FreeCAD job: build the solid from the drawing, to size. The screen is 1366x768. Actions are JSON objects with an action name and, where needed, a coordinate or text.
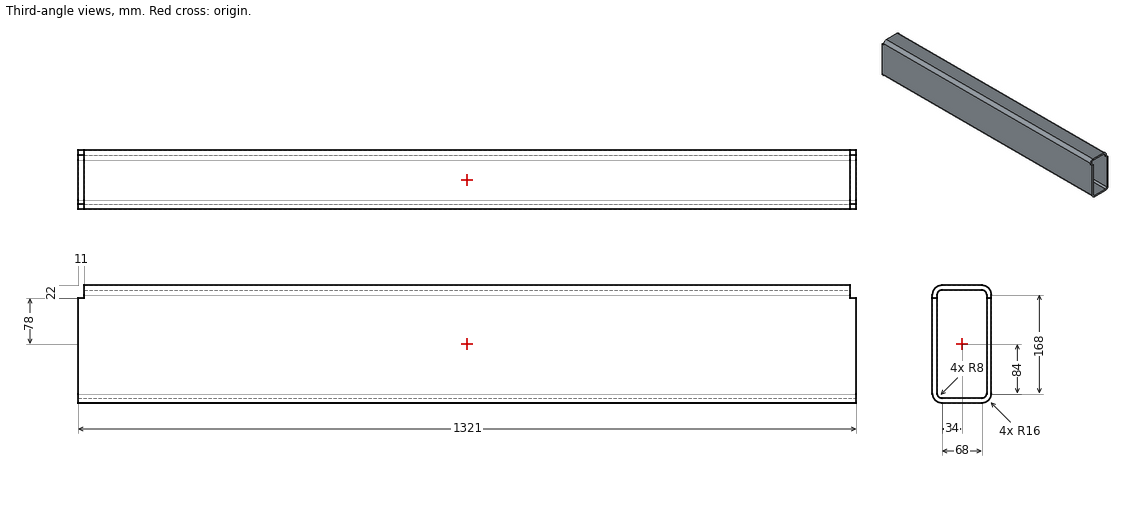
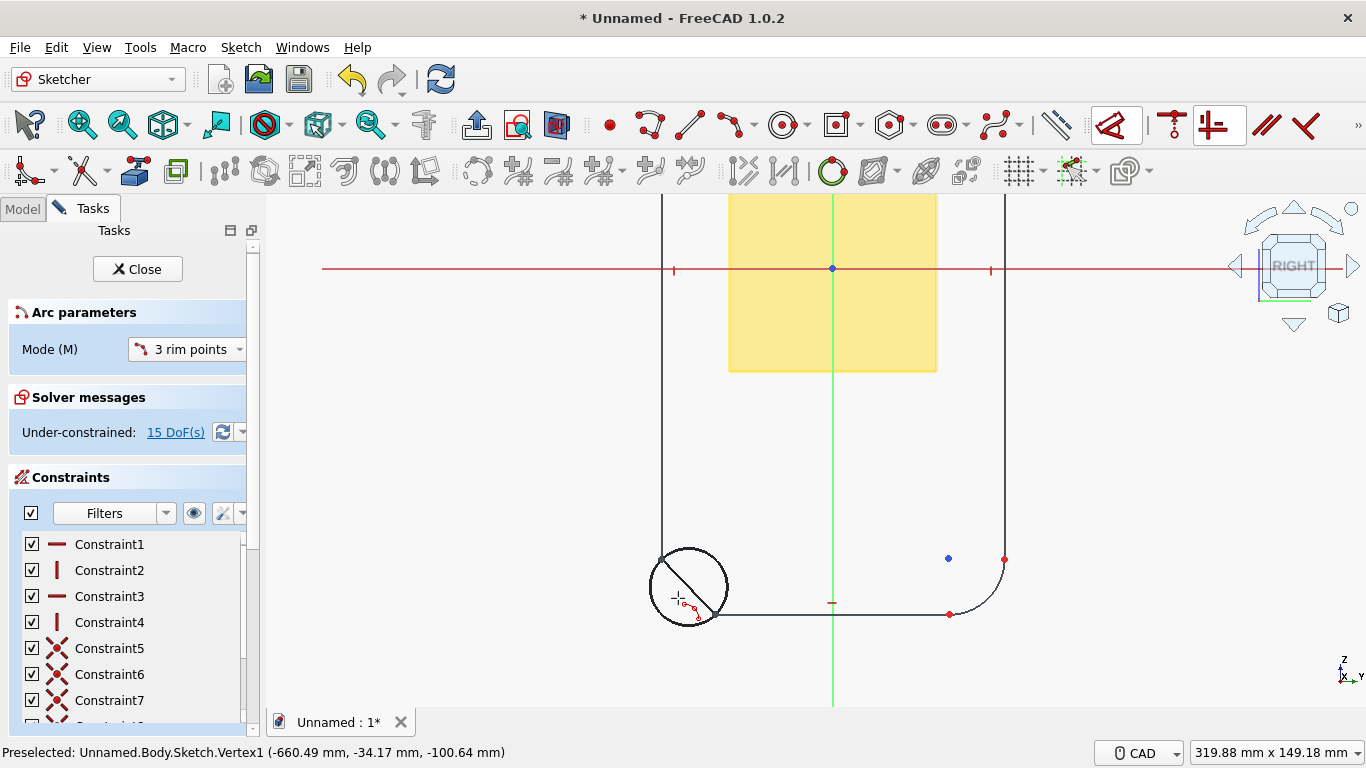
{"action": "left_click", "coordinate": [677, 597]}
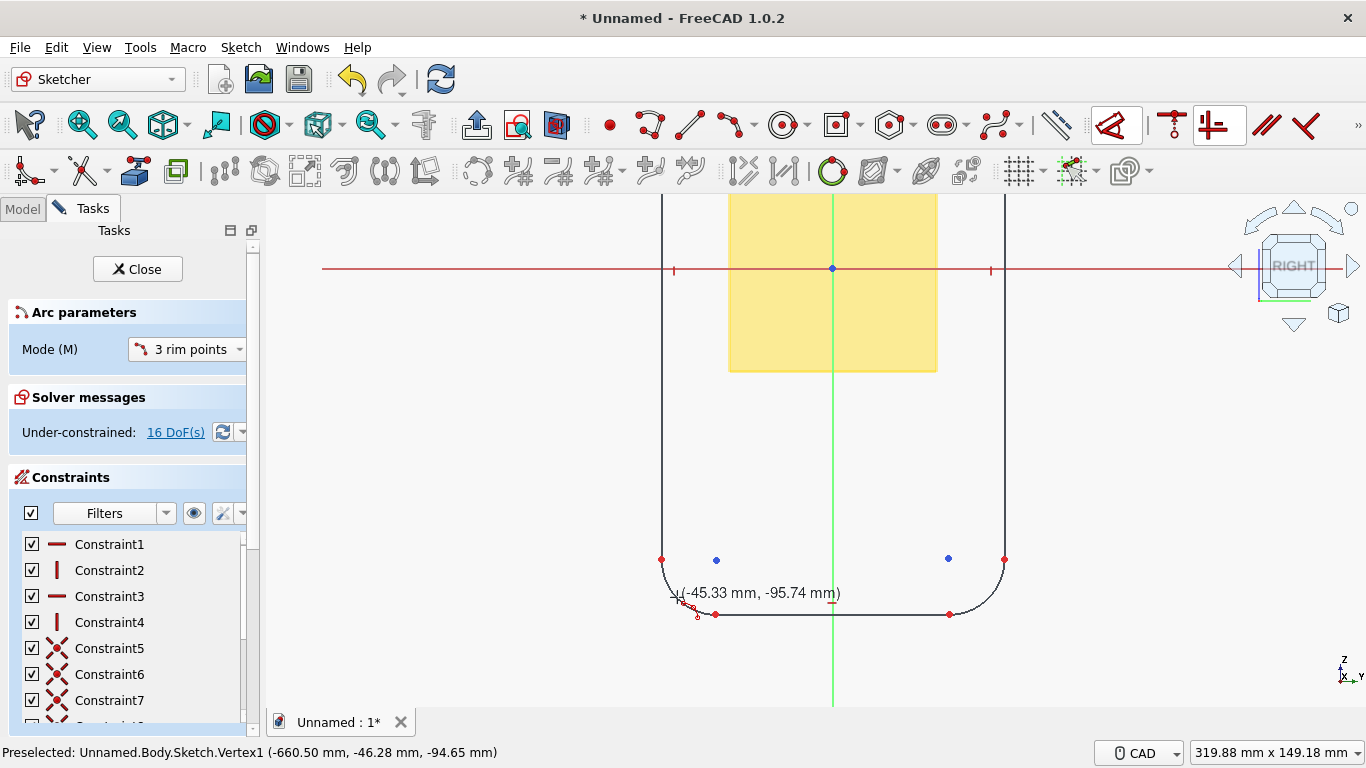
{"action": "key", "text": "g l"}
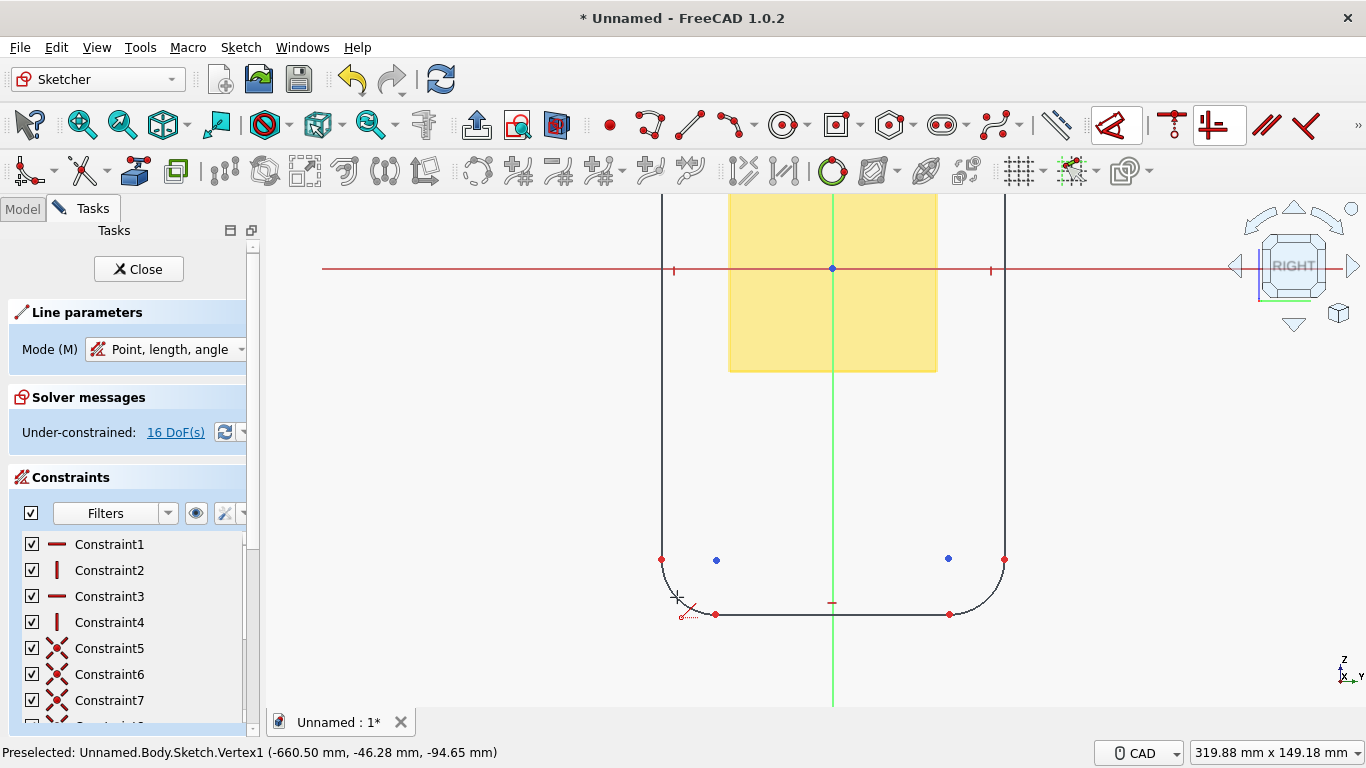
{"action": "left_click", "coordinate": [950, 585]}
{"action": "left_click", "coordinate": [716, 585]}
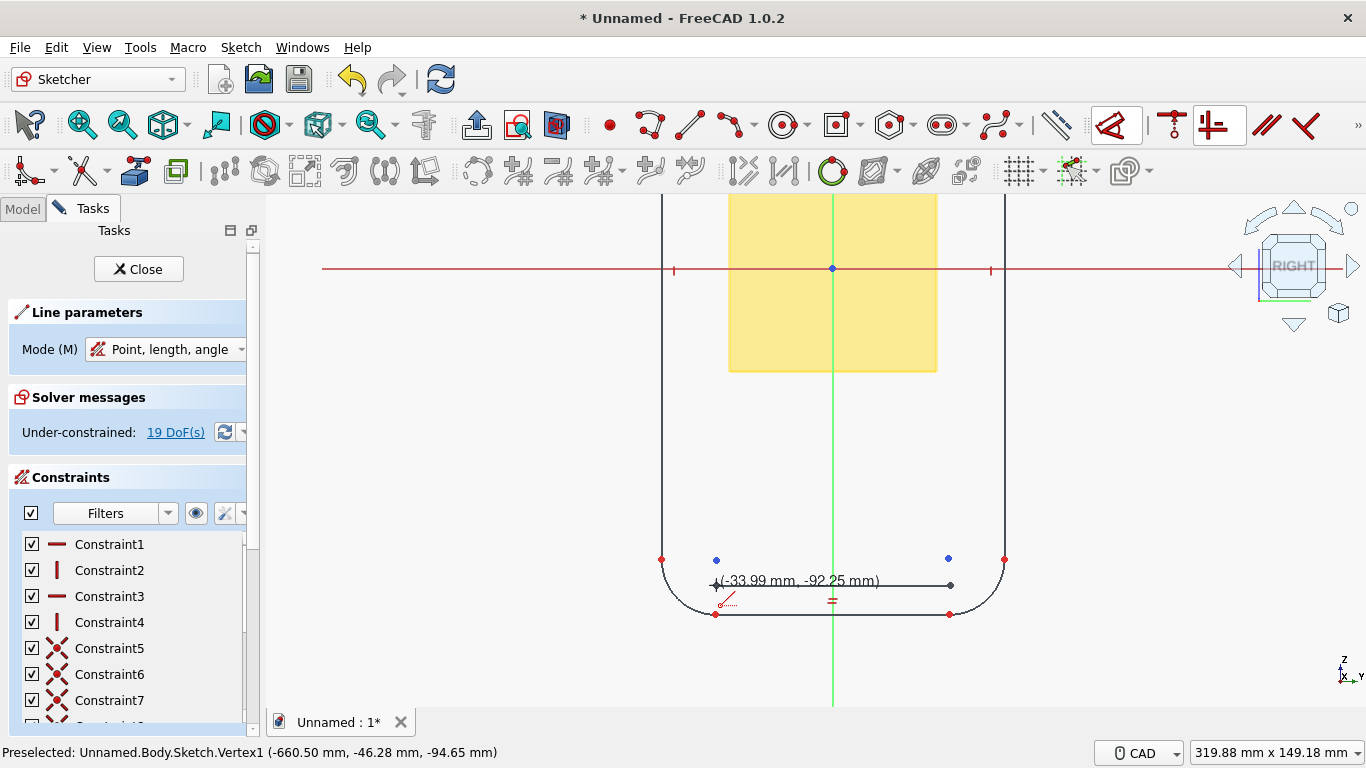
{"action": "left_click", "coordinate": [688, 558]}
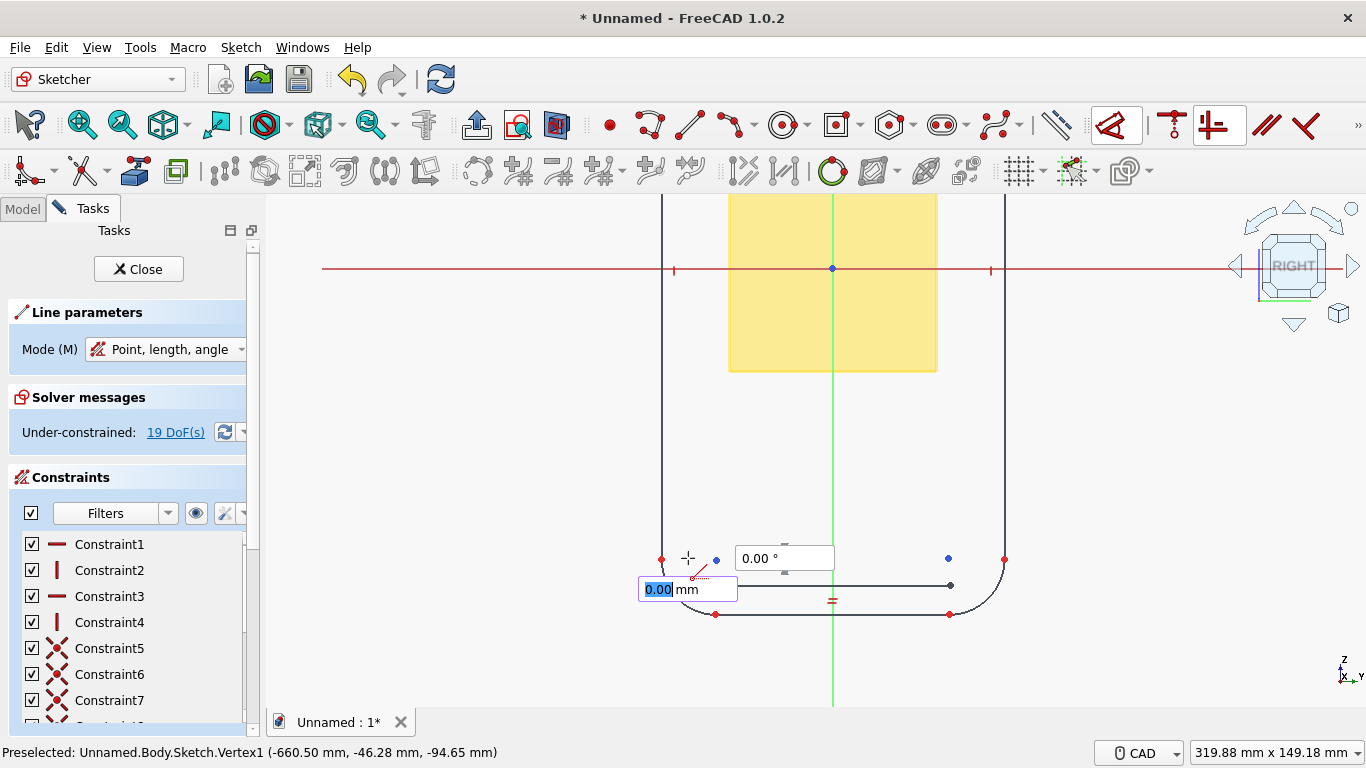
{"action": "scroll", "coordinate": [678, 599], "scroll_direction": "down", "scroll_amount": 4}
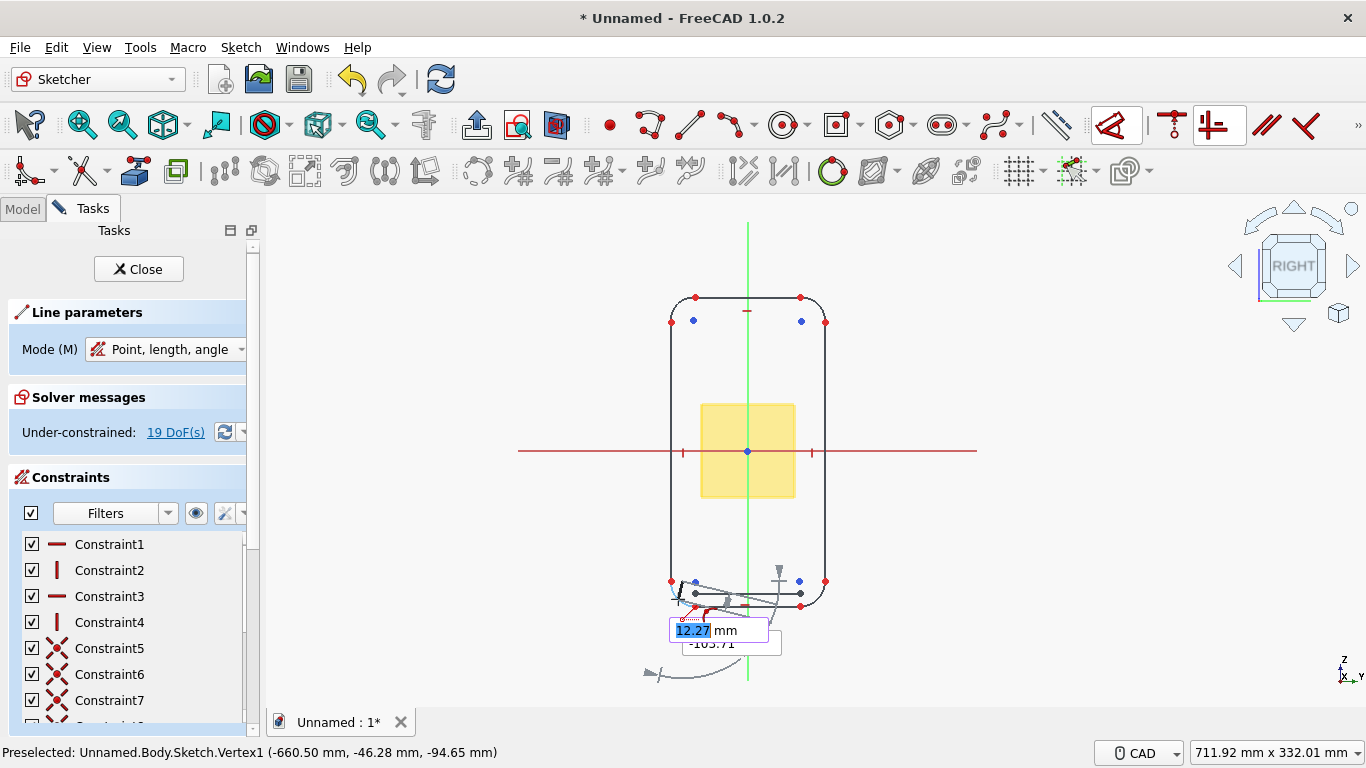
{"action": "scroll", "coordinate": [683, 321], "scroll_direction": "up", "scroll_amount": 2}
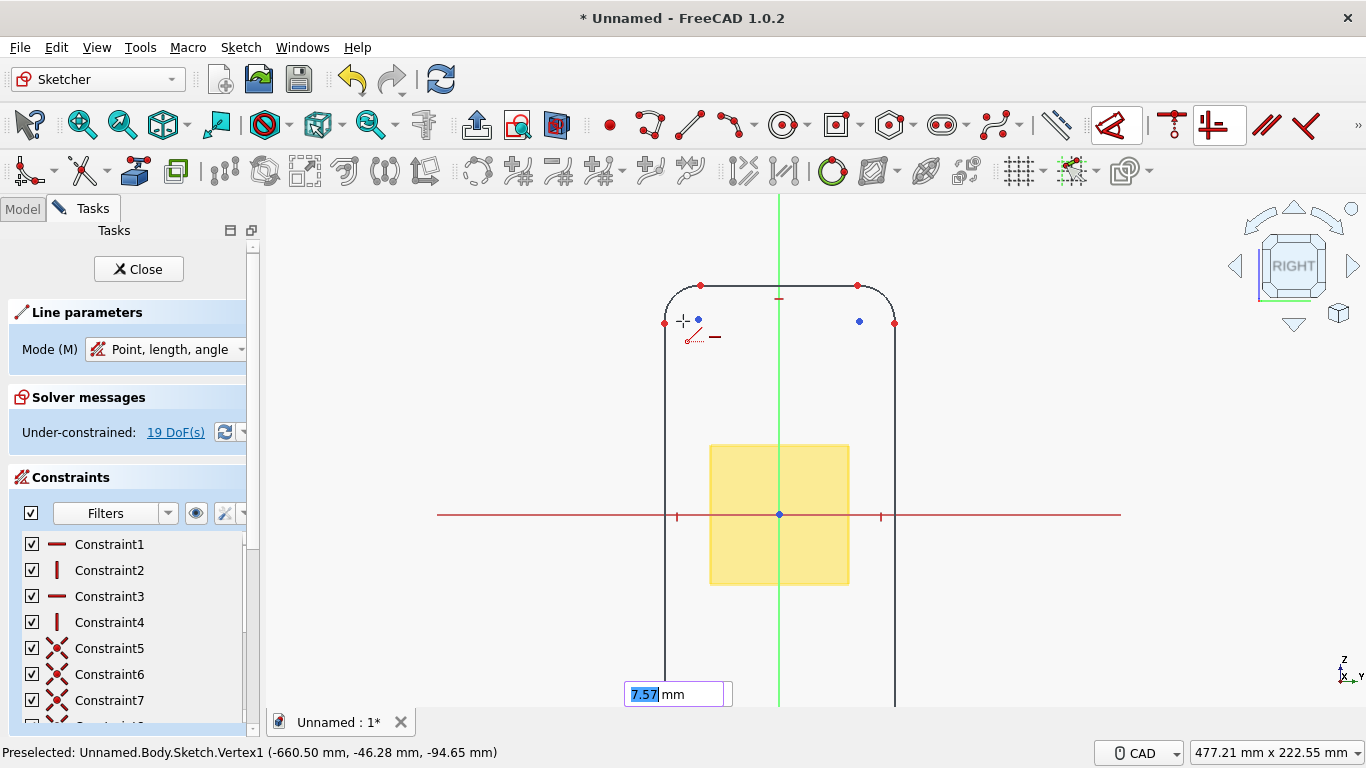
{"action": "left_click", "coordinate": [682, 321]}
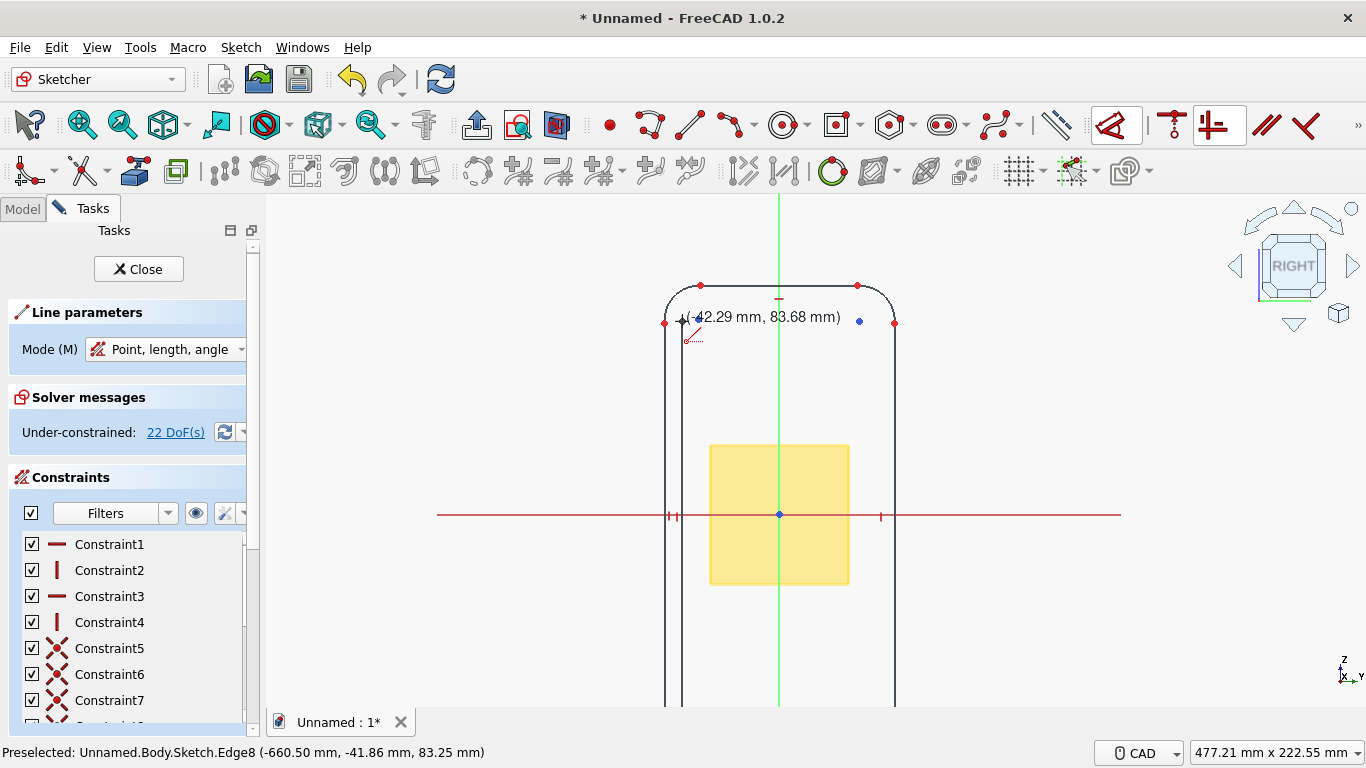
{"action": "left_click", "coordinate": [701, 303]}
{"action": "left_click", "coordinate": [858, 303]}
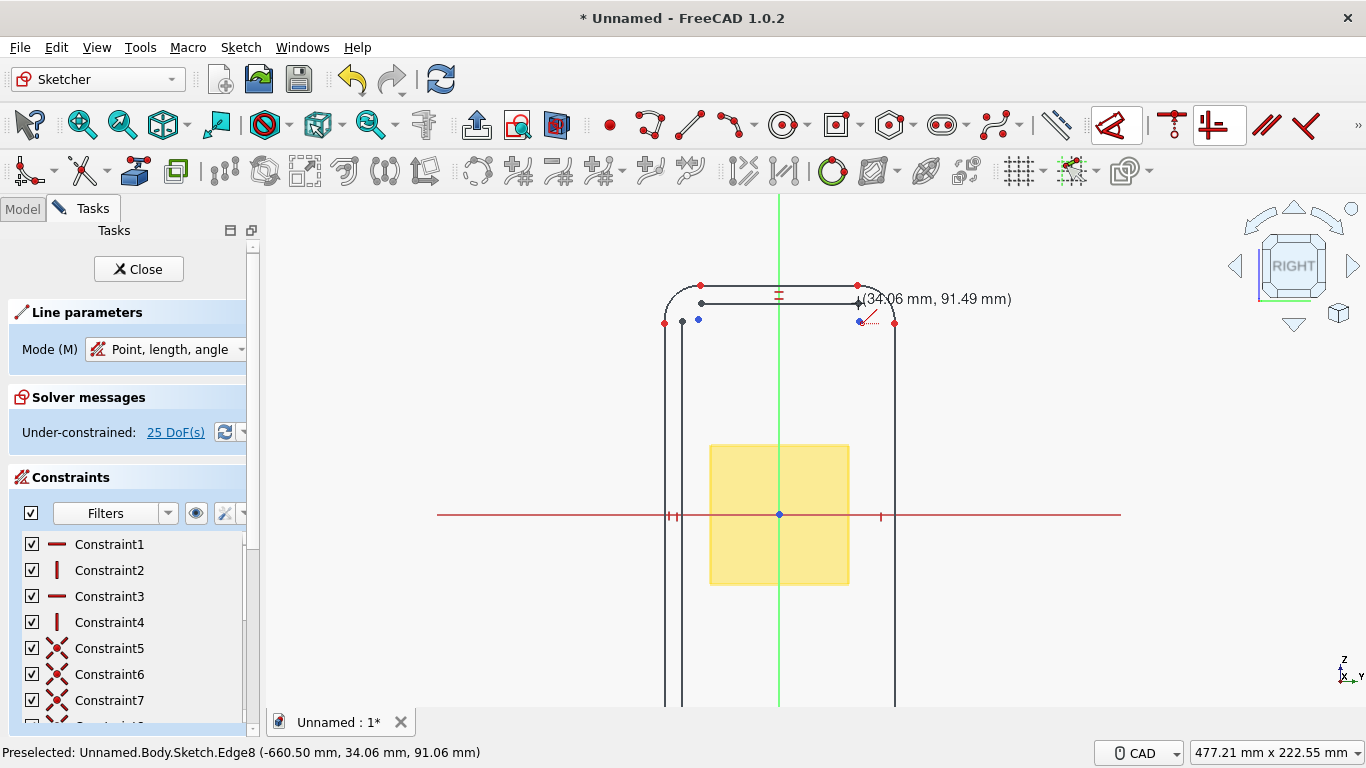
{"action": "left_click", "coordinate": [876, 321]}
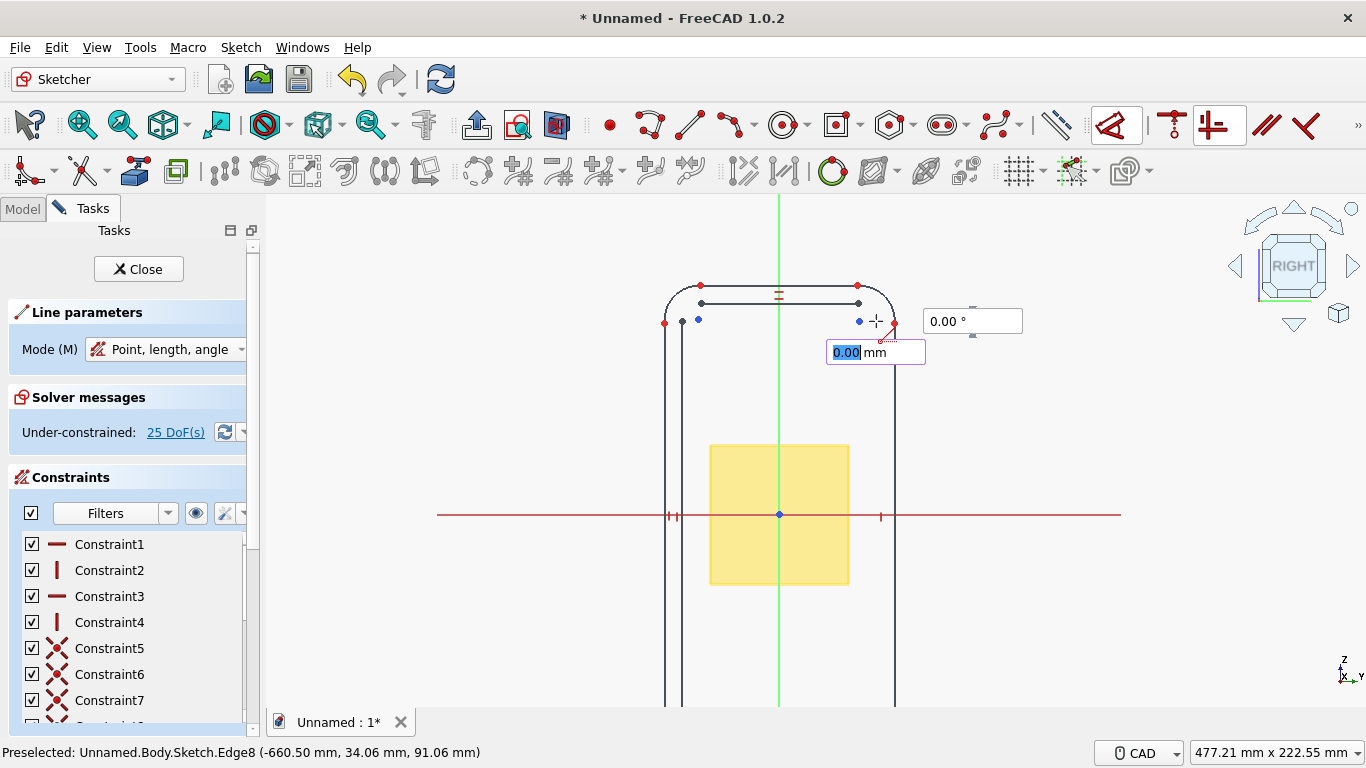
{"action": "scroll", "coordinate": [682, 320], "scroll_direction": "down", "scroll_amount": 2}